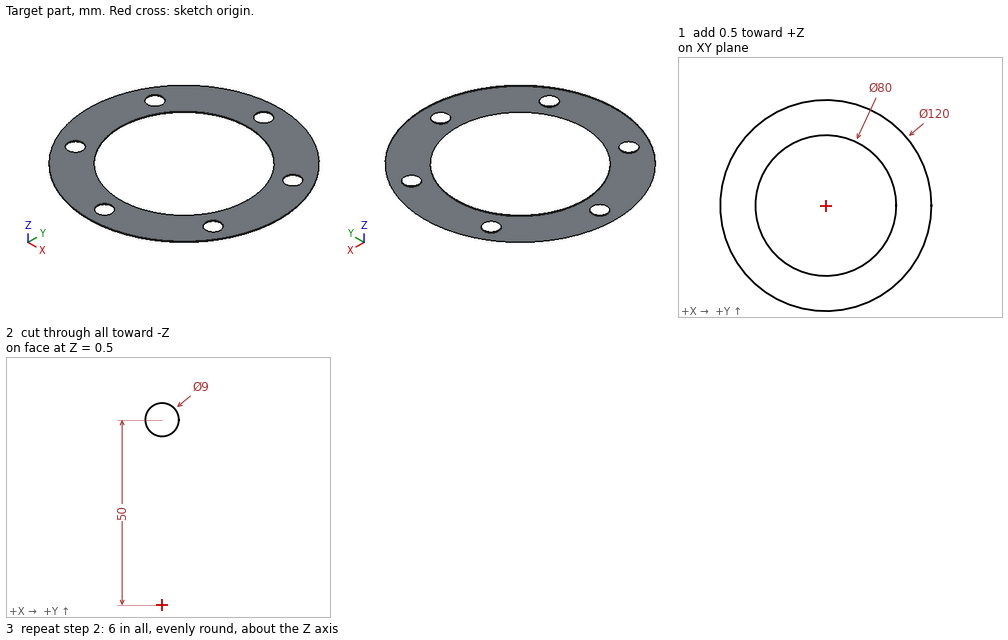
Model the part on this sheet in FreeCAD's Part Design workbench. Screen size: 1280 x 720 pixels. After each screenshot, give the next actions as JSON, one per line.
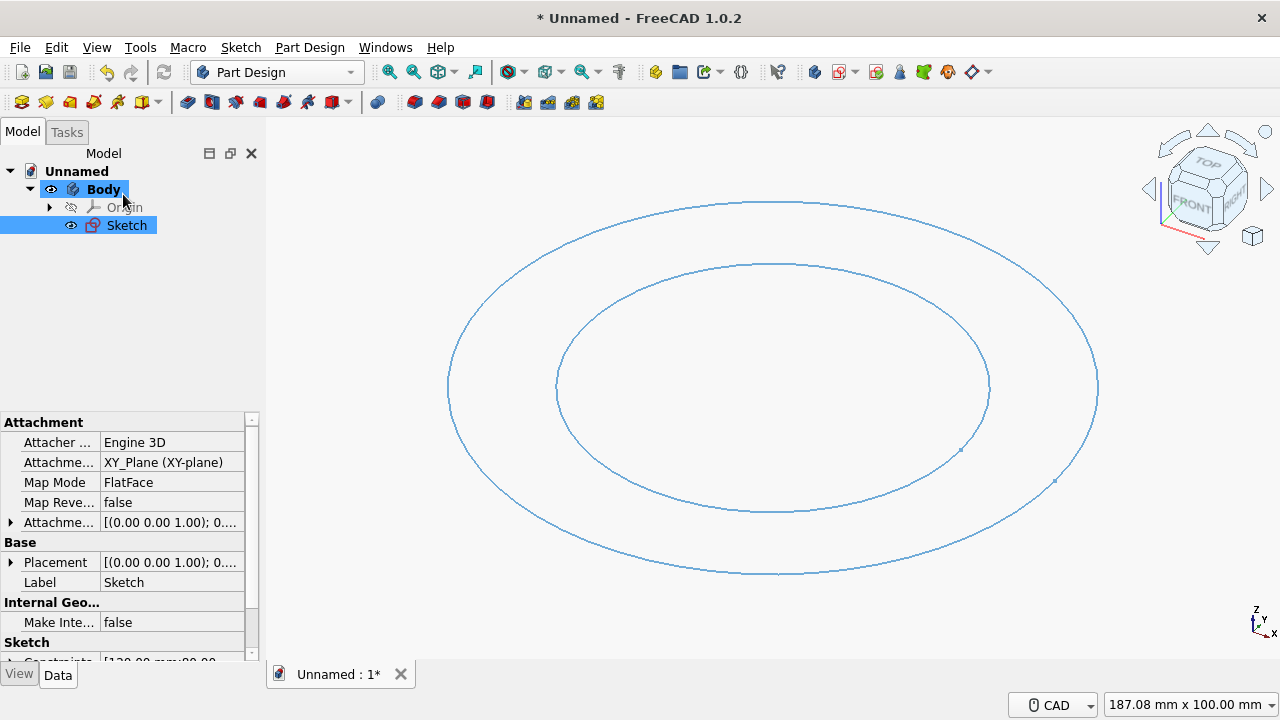
{"action": "left_click", "coordinate": [22, 102]}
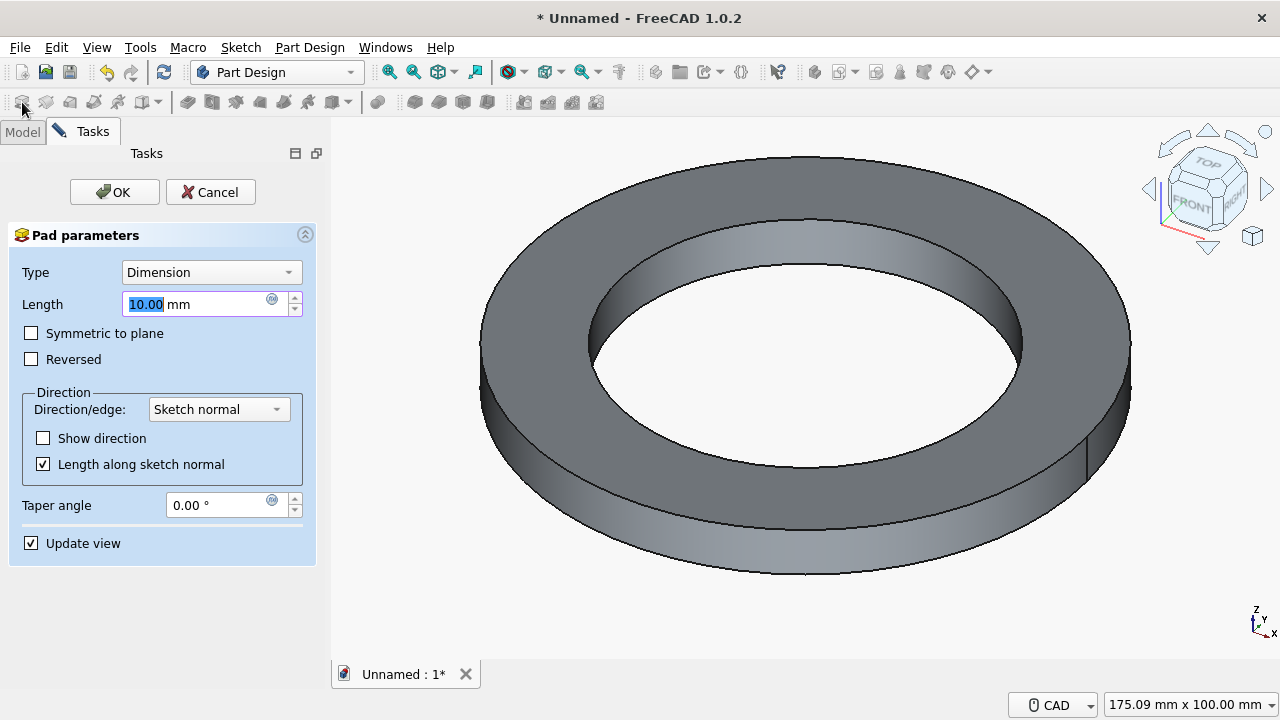
{"action": "type", "text": "0.5"}
{"action": "key", "text": "Tab"}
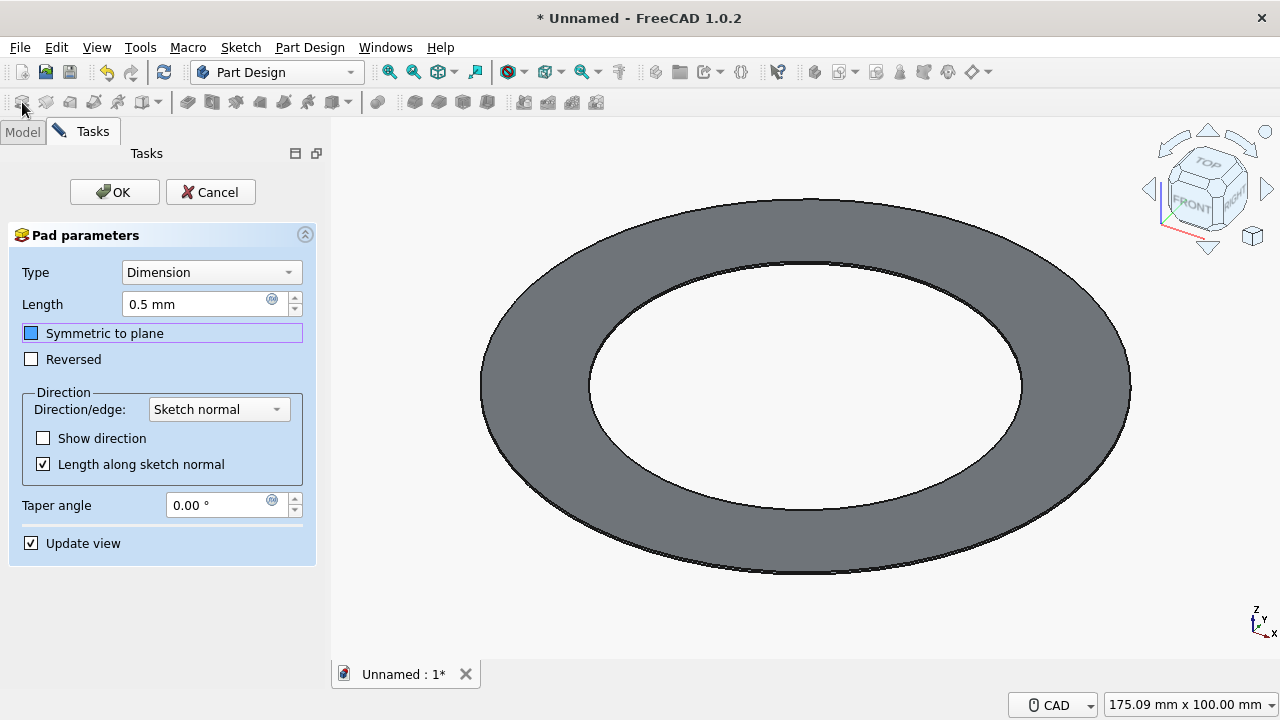
{"action": "left_click", "coordinate": [115, 192]}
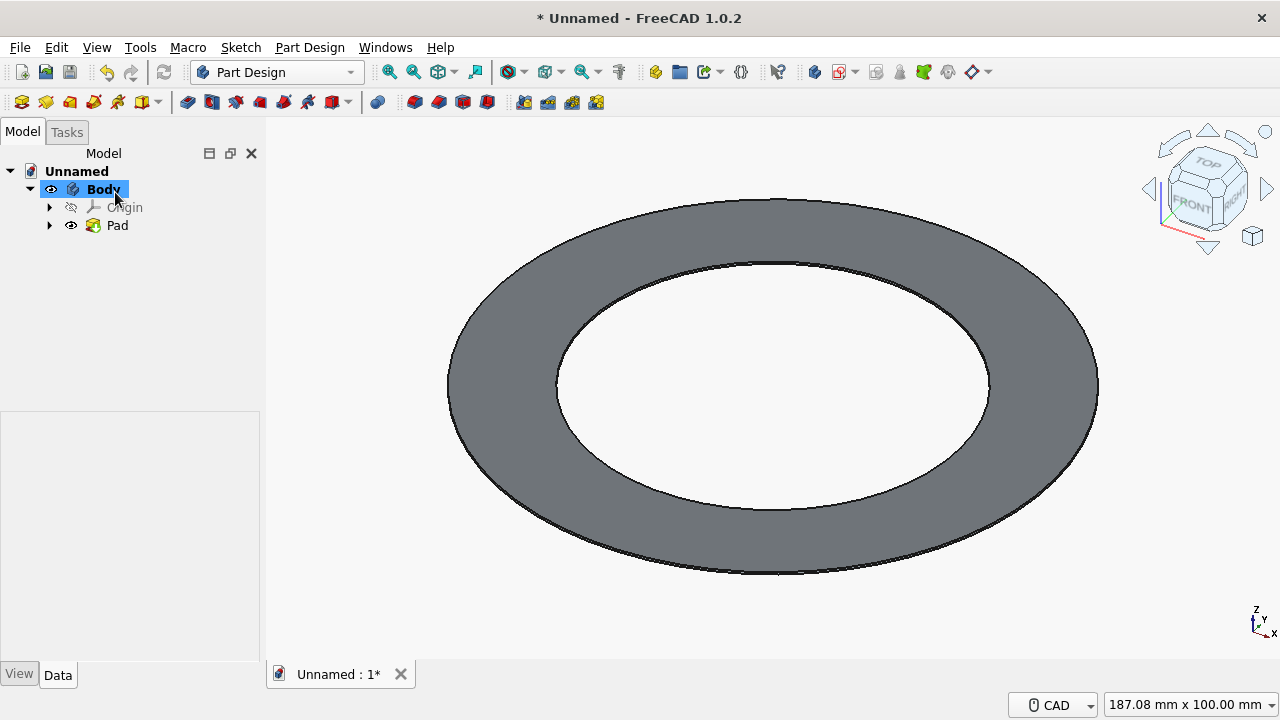
{"action": "left_click", "coordinate": [1014, 465]}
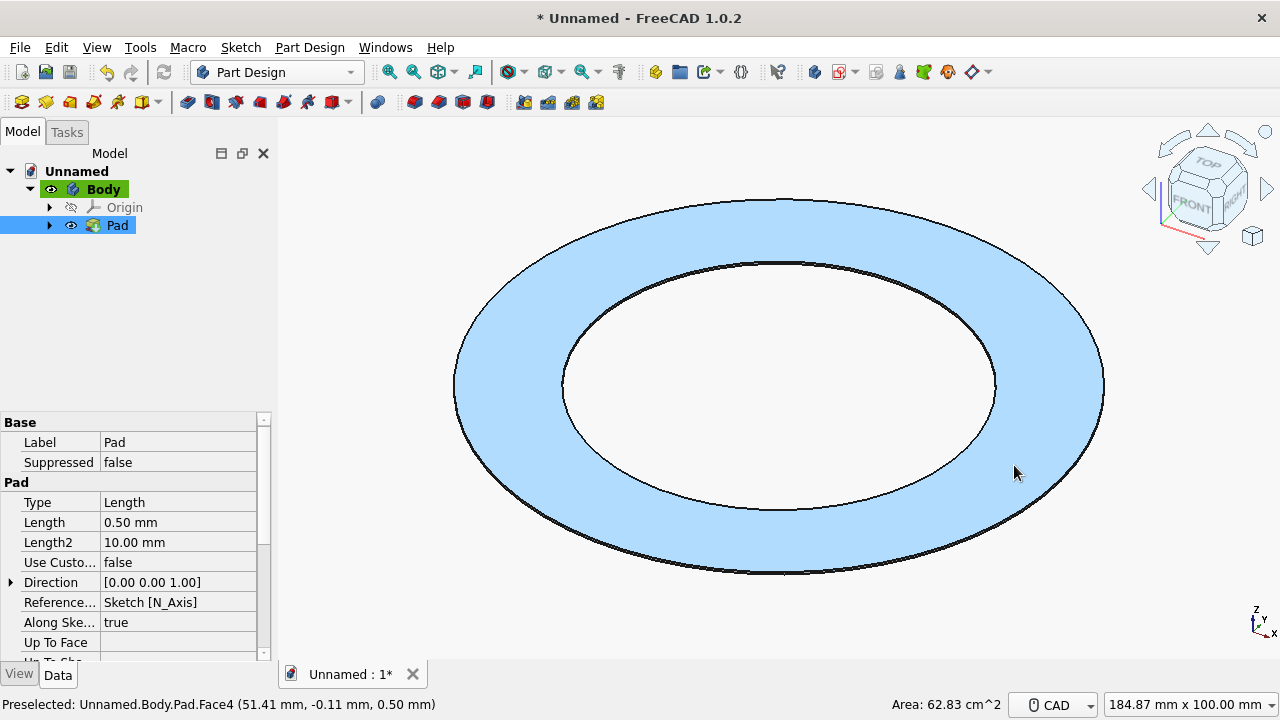
{"action": "left_click", "coordinate": [840, 72]}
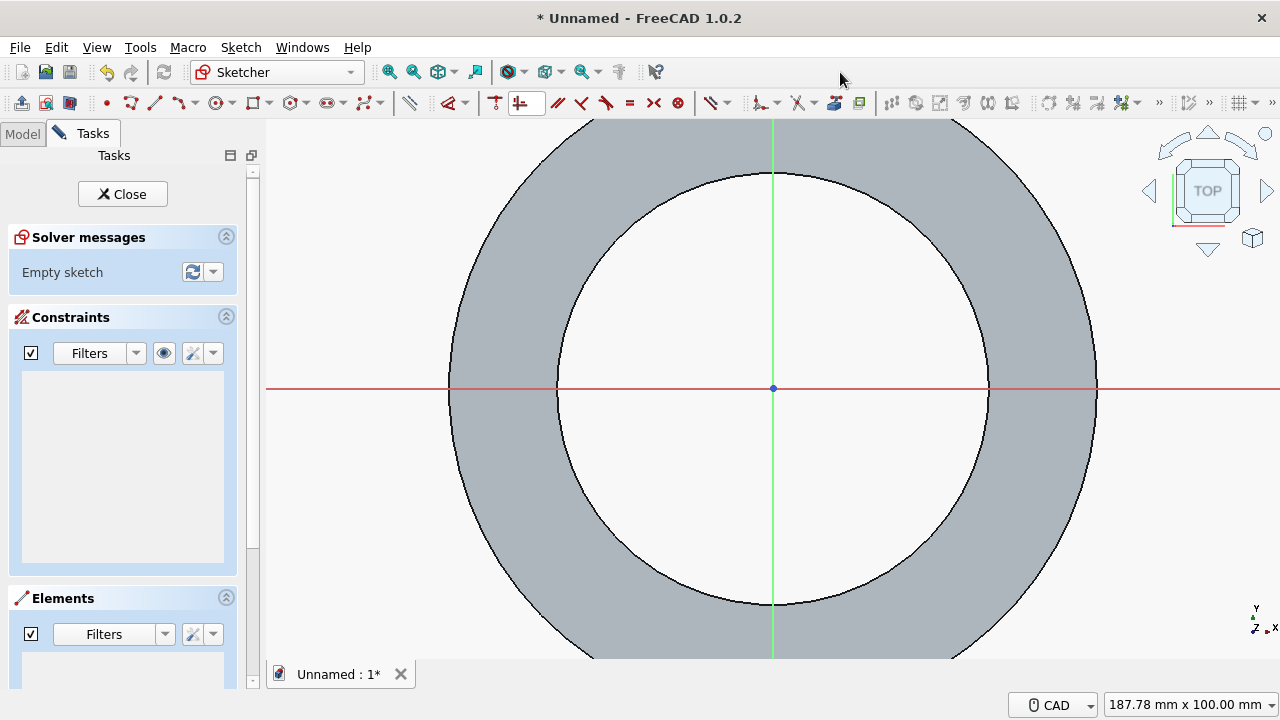
{"action": "scroll", "coordinate": [704, 389], "scroll_direction": "down", "scroll_amount": 5}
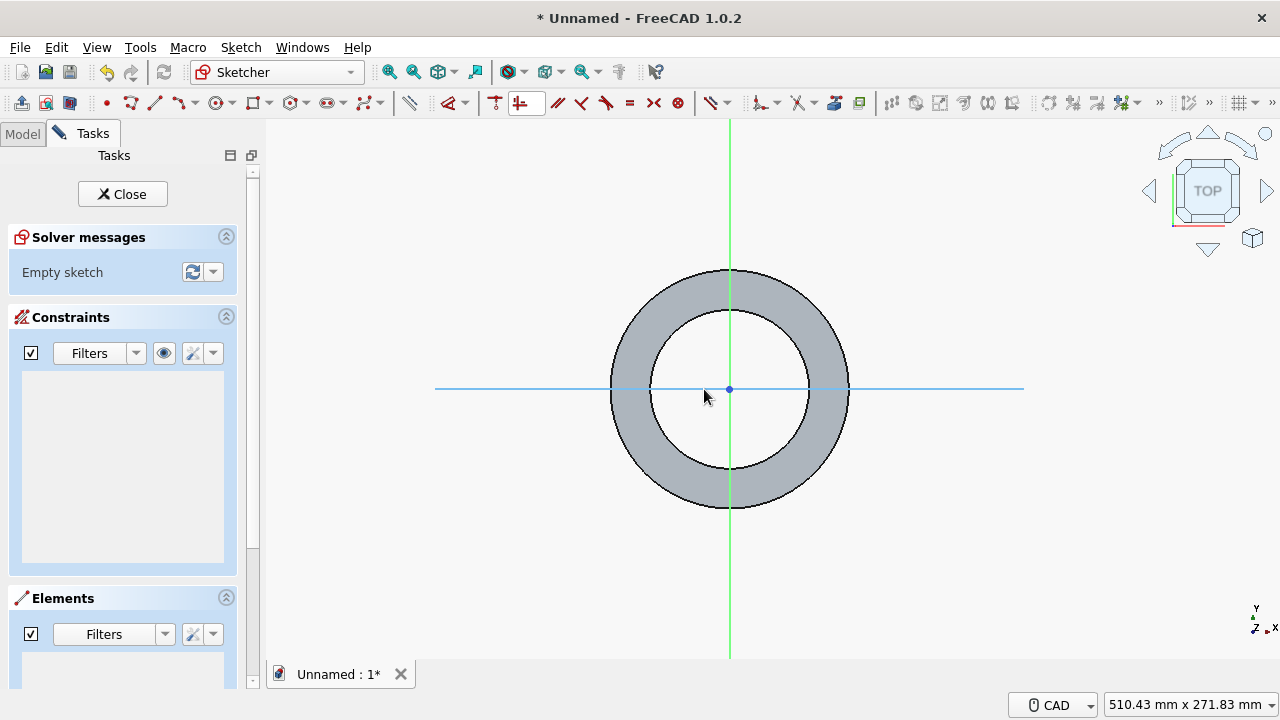
{"action": "scroll", "coordinate": [731, 285], "scroll_direction": "up", "scroll_amount": 15}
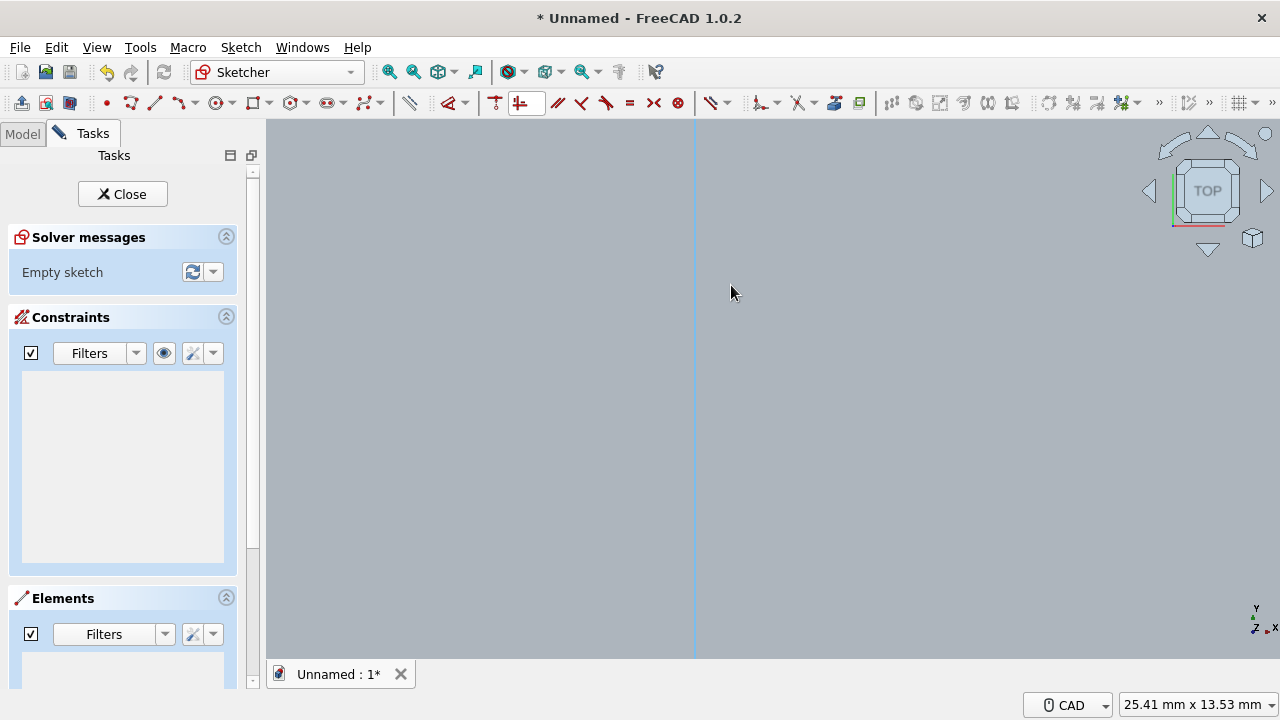
{"action": "left_click", "coordinate": [216, 104]}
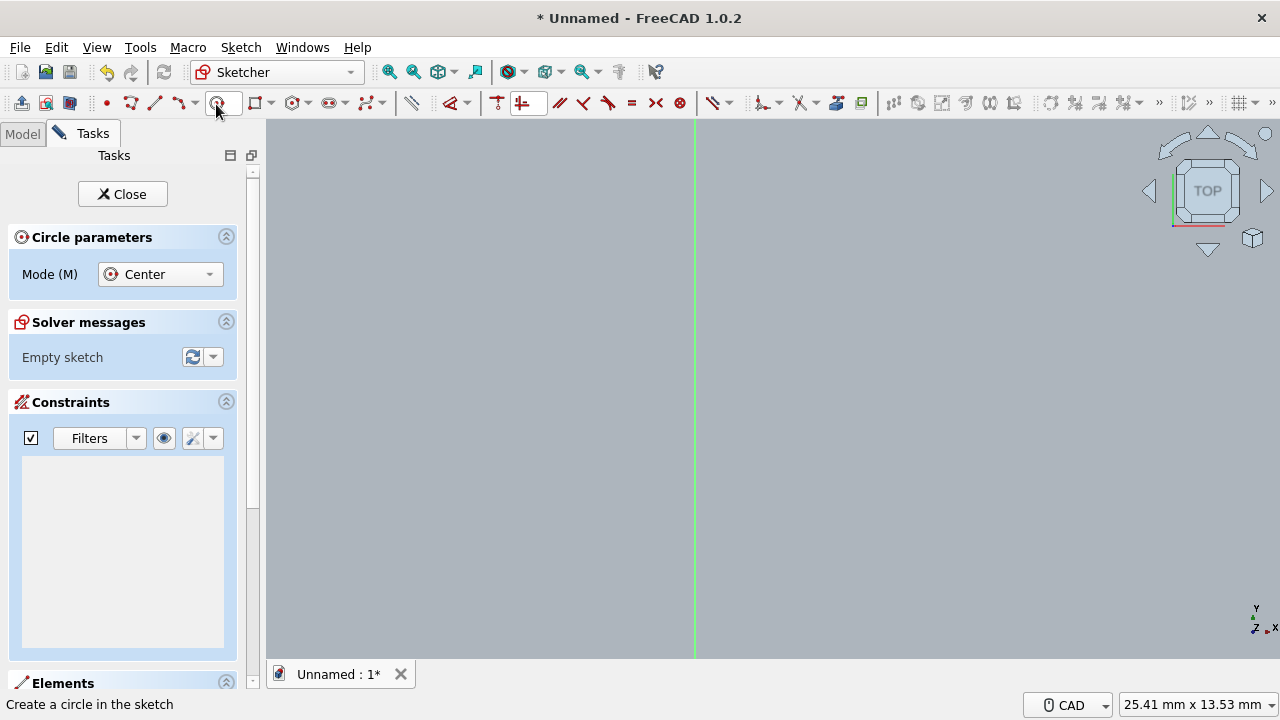
{"action": "left_click", "coordinate": [695, 379]}
{"action": "mouse_move", "coordinate": [822, 252]}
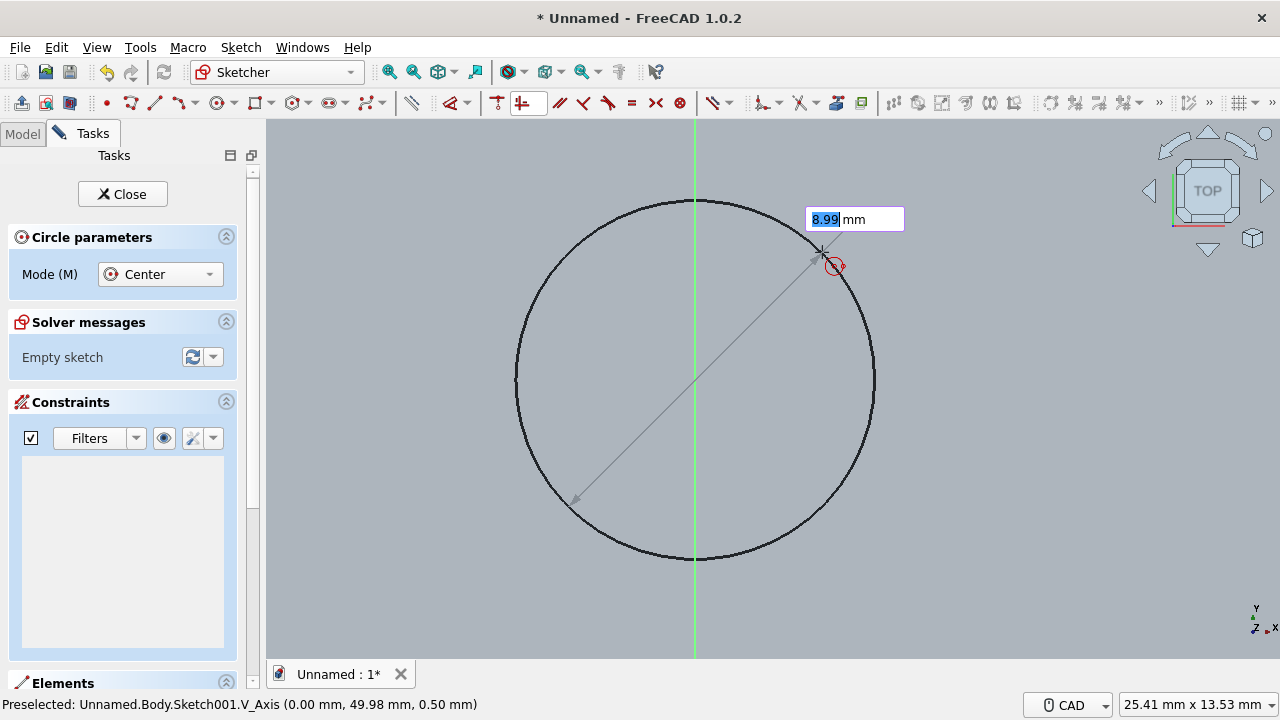
{"action": "type", "text": "9"}
{"action": "key", "text": "Return"}
{"action": "key", "text": "Escape"}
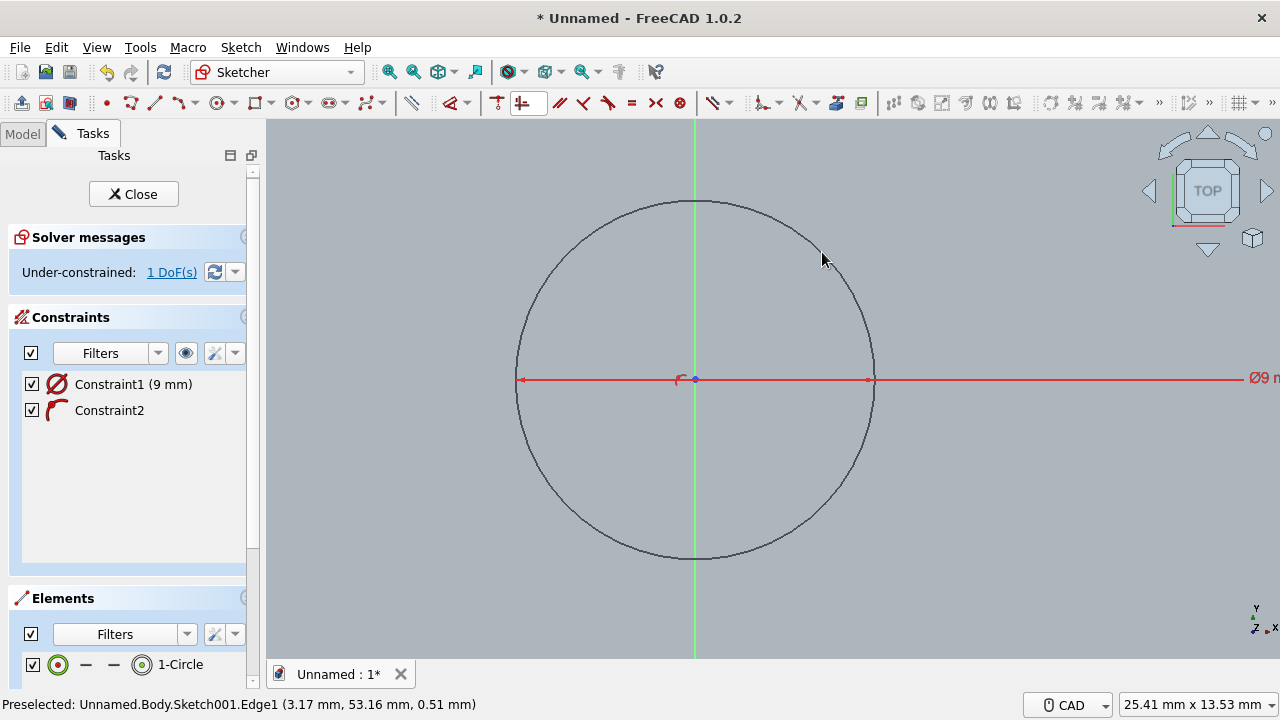
{"action": "left_click", "coordinate": [450, 104]}